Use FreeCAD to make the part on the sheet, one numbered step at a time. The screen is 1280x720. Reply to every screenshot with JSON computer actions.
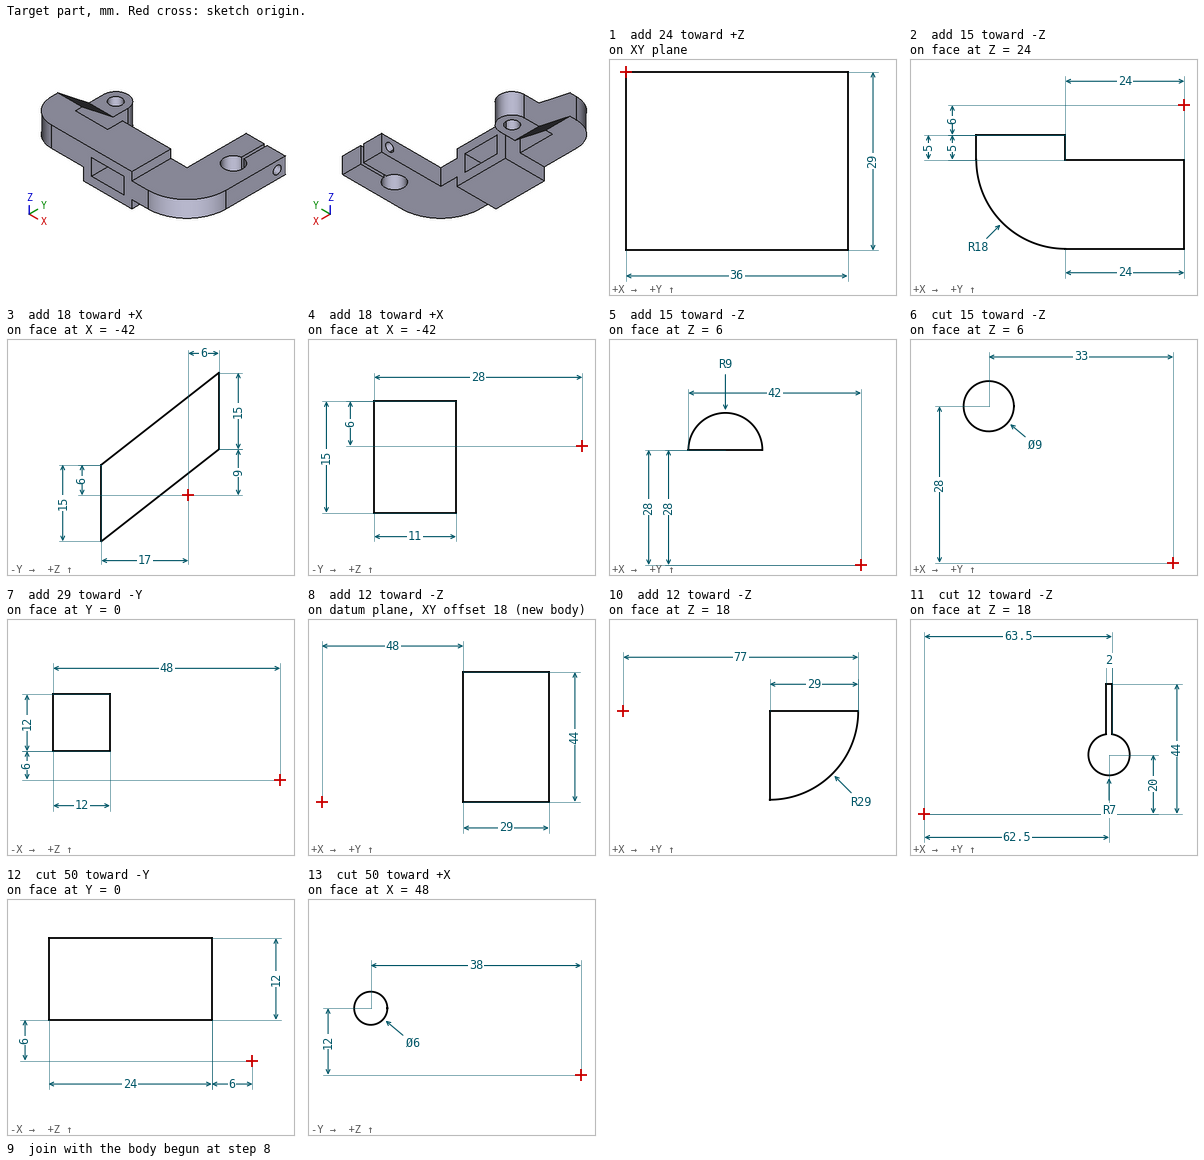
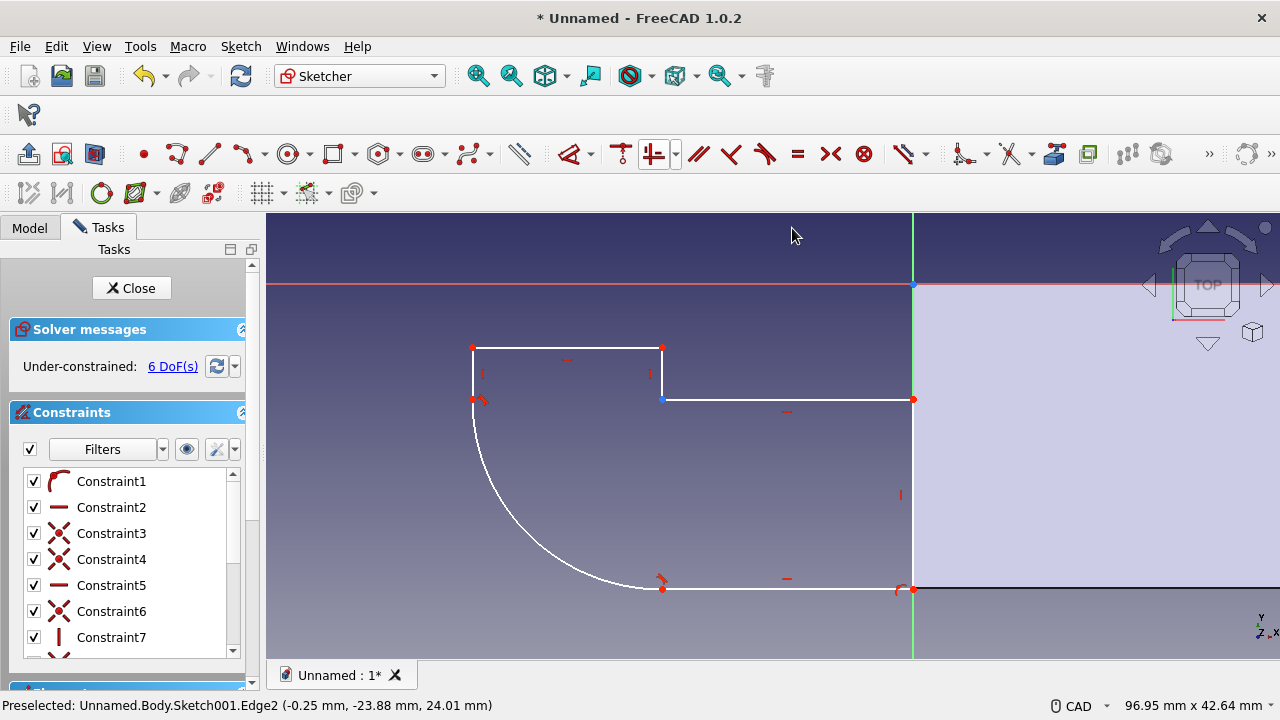
{"action": "left_click", "coordinate": [493, 486]}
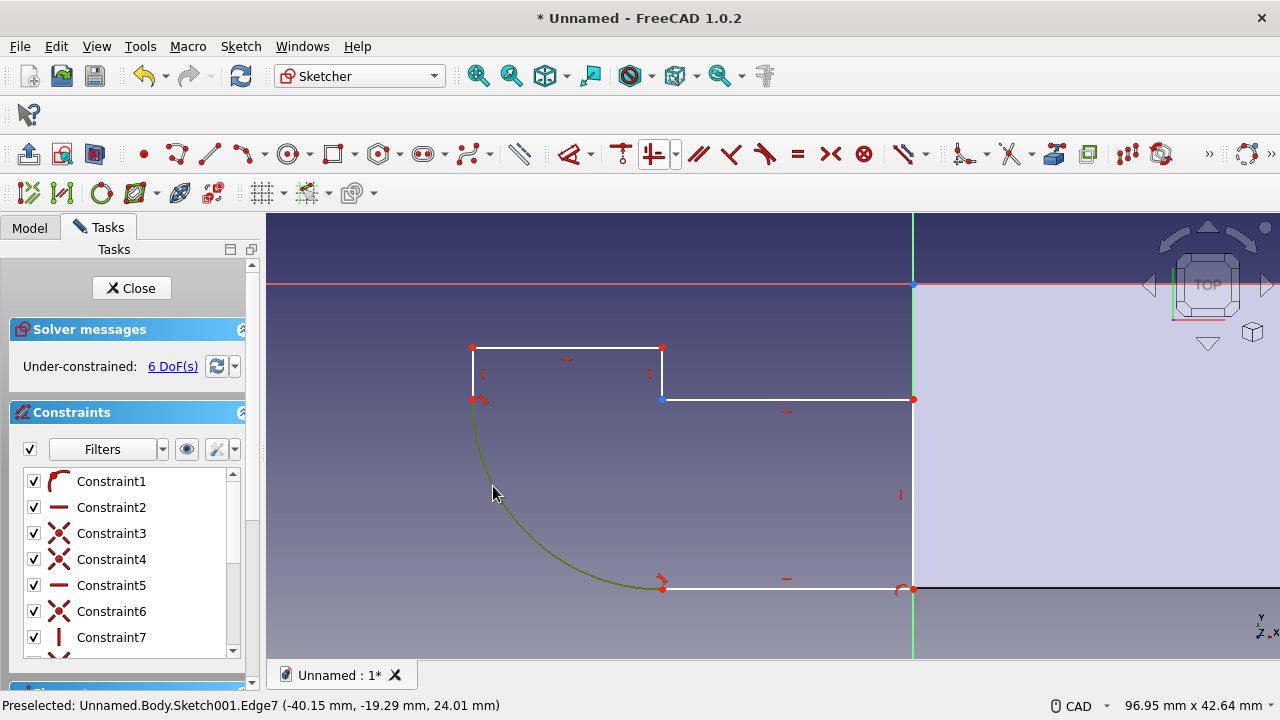
{"action": "key", "text": "k r"}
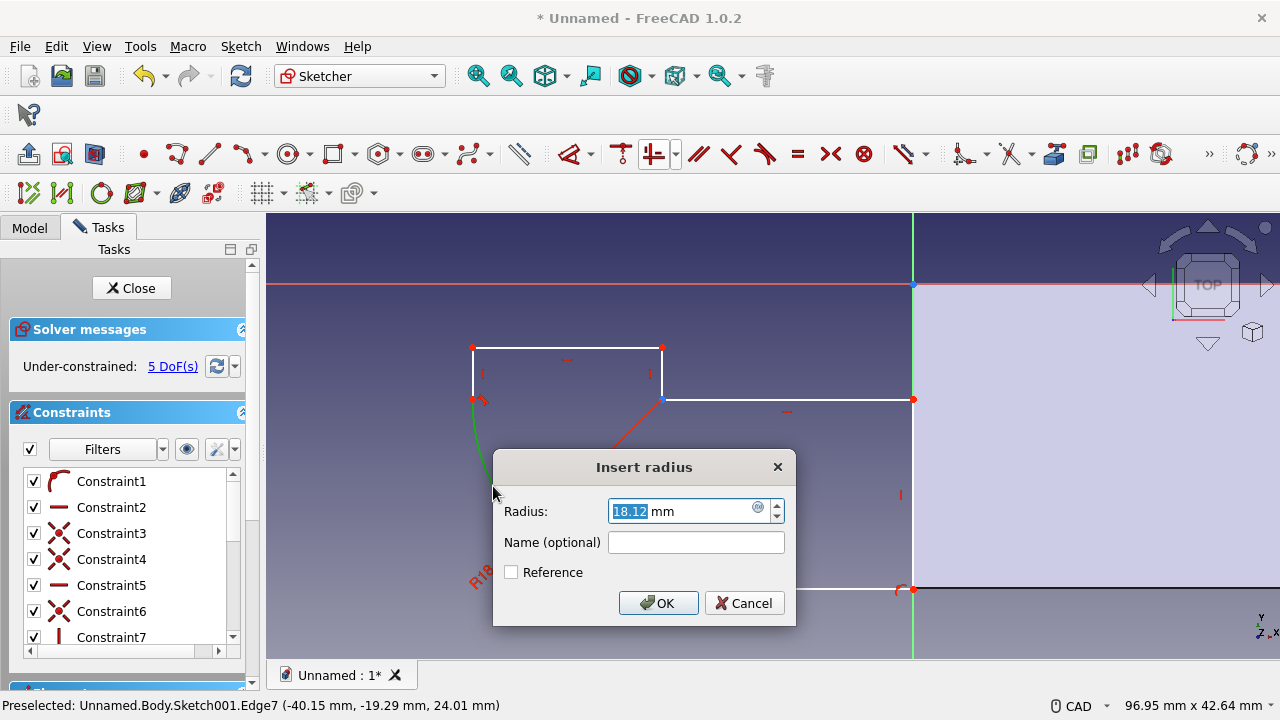
{"action": "type", "text": "18"}
{"action": "key", "text": "Return"}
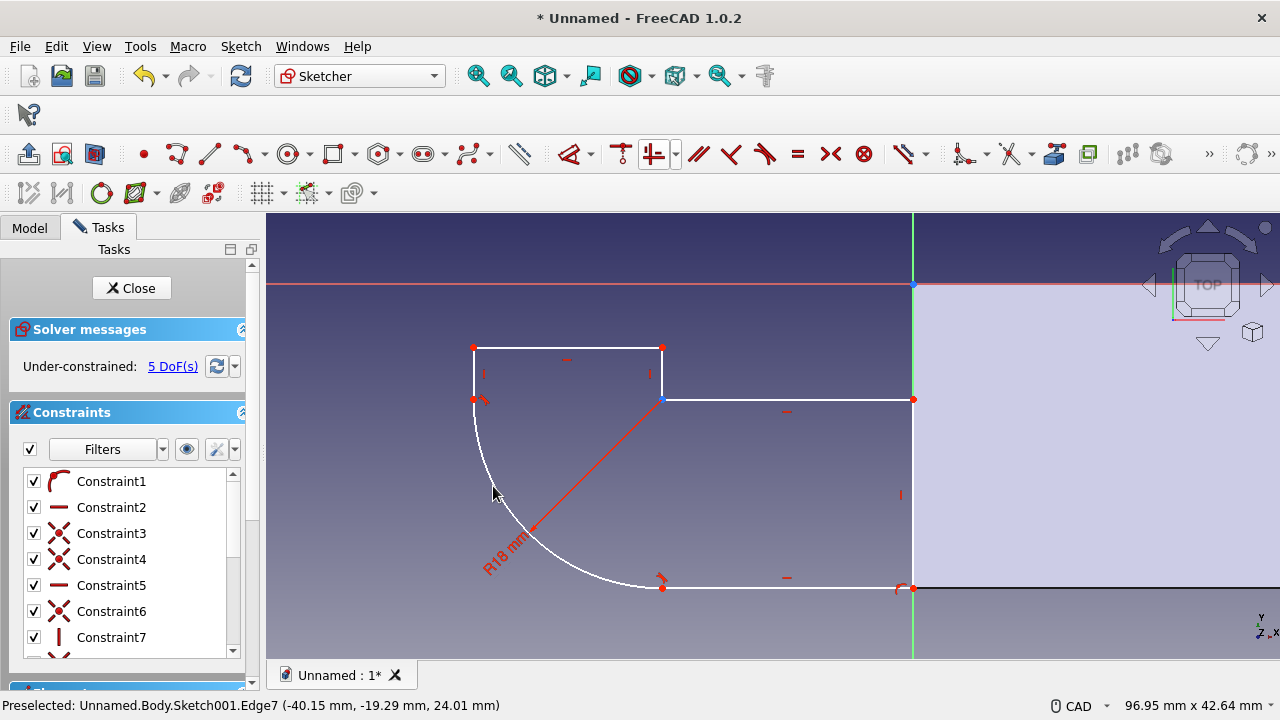
{"action": "left_click", "coordinate": [662, 384]}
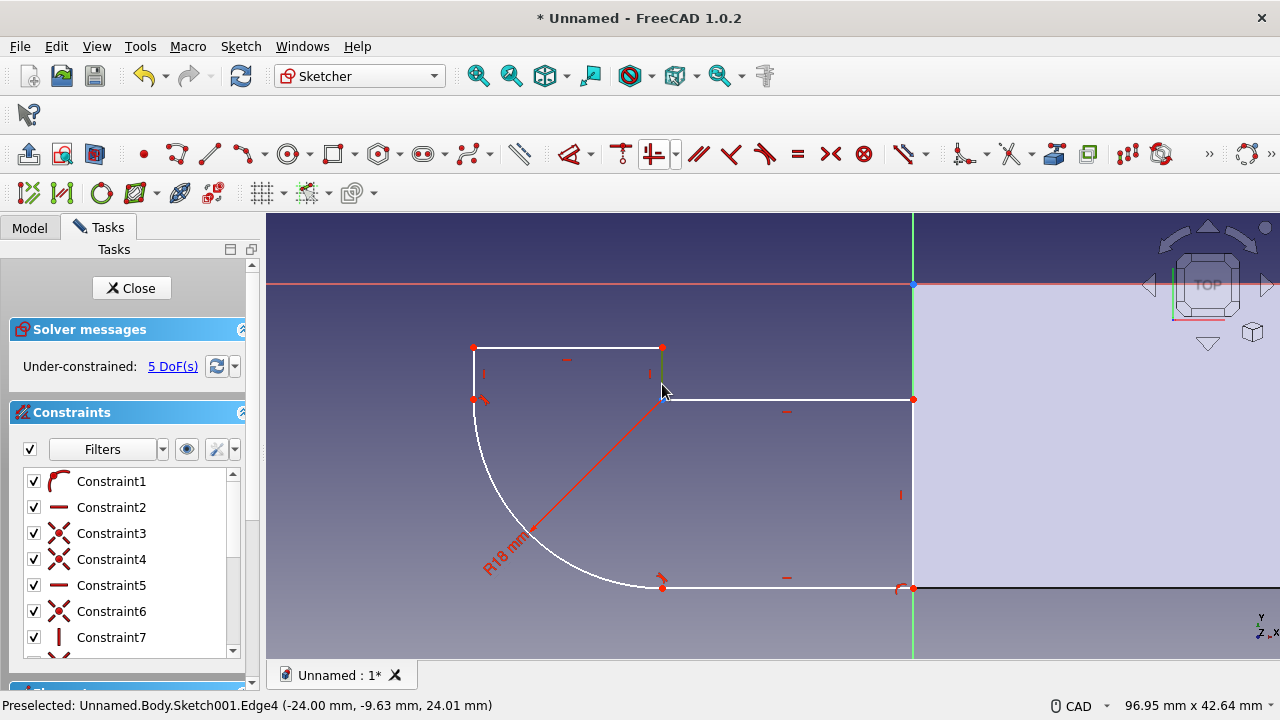
{"action": "key", "text": "i"}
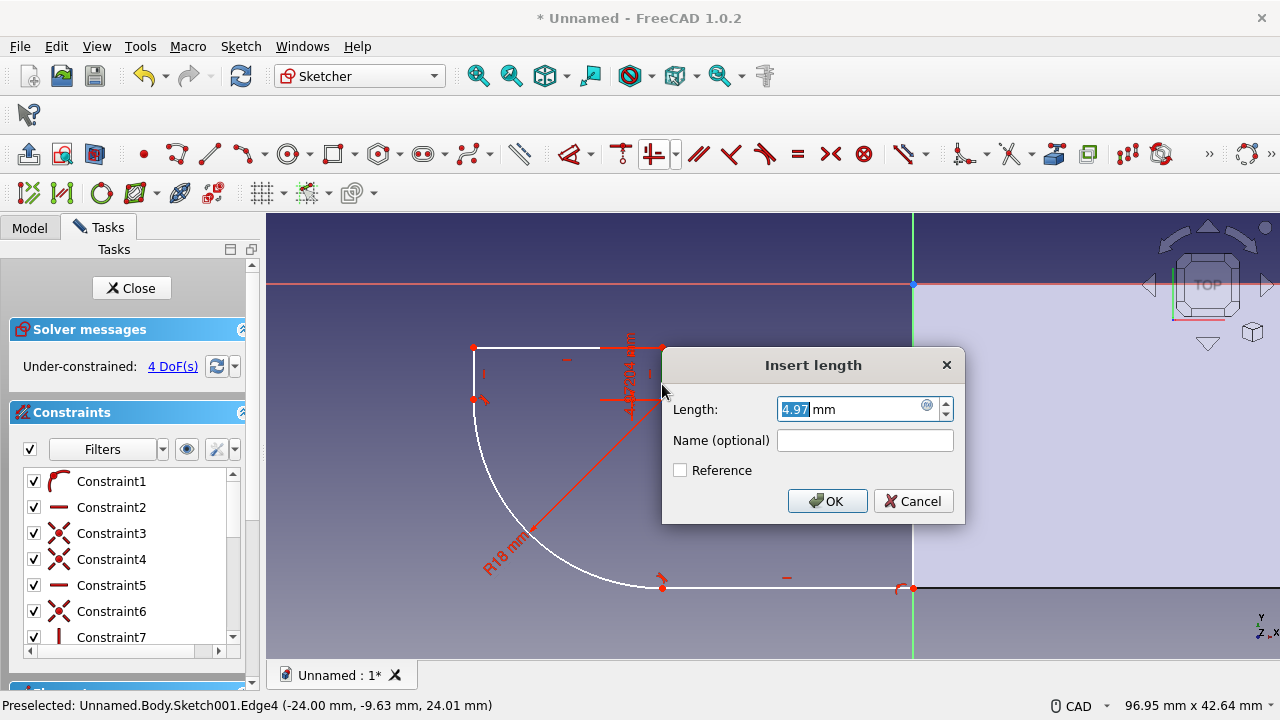
{"action": "type", "text": "5"}
{"action": "key", "text": "Return"}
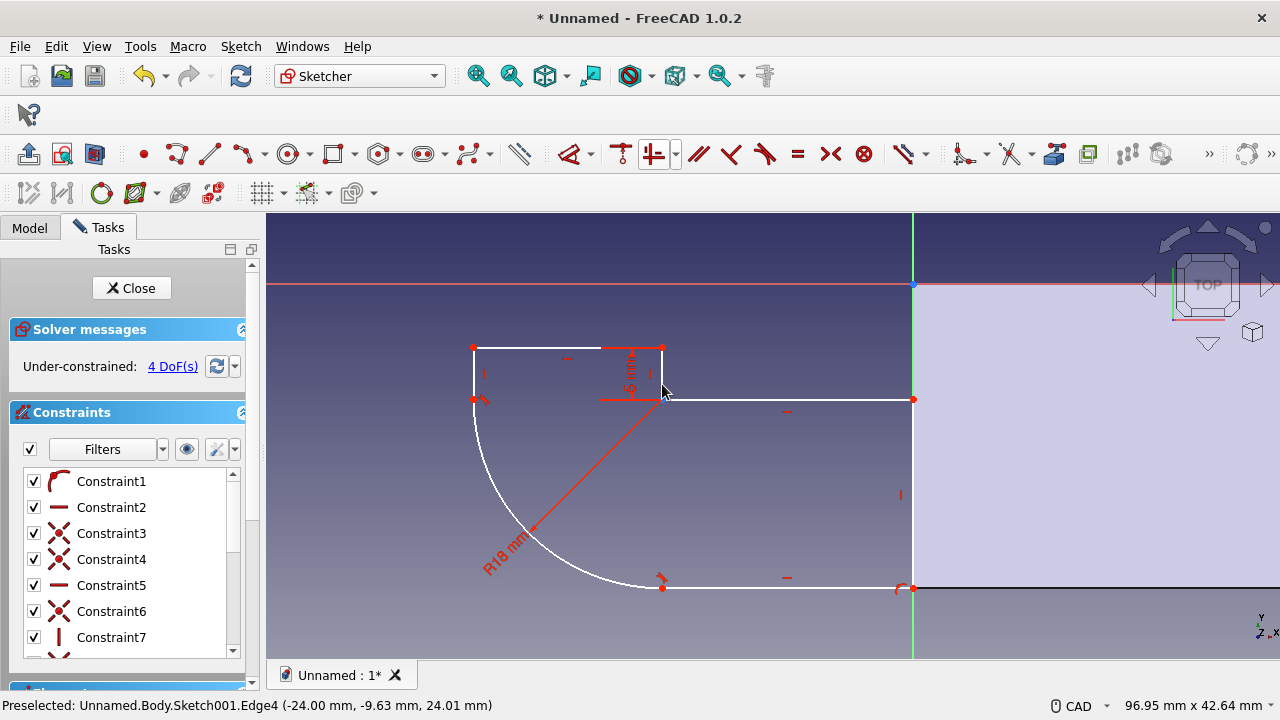
{"action": "left_click", "coordinate": [474, 363]}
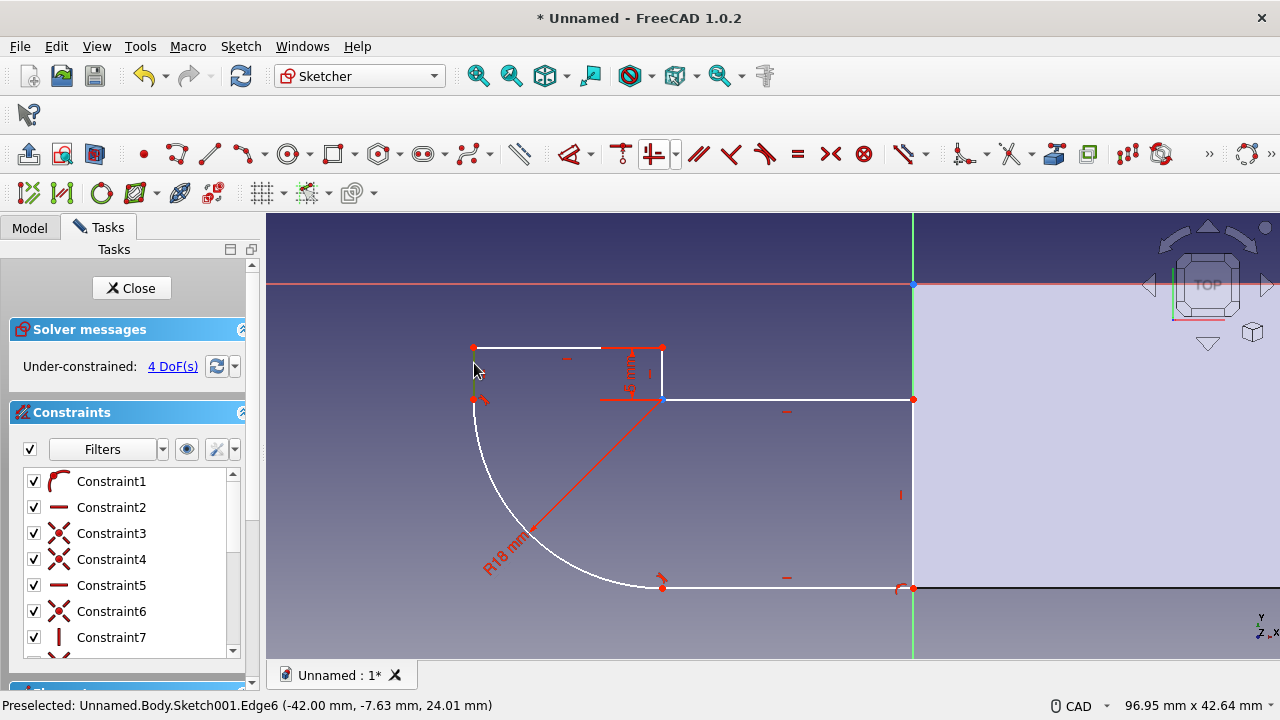
{"action": "key", "text": "i"}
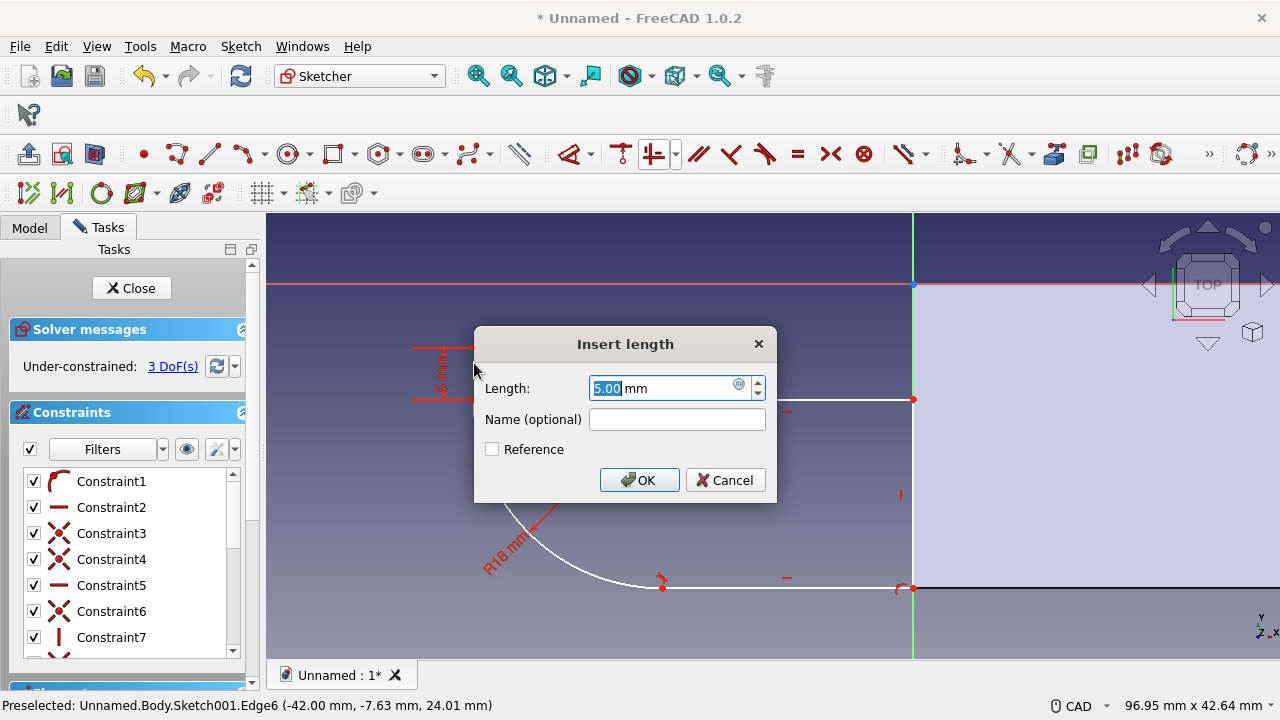
{"action": "type", "text": "5"}
{"action": "key", "text": "Return"}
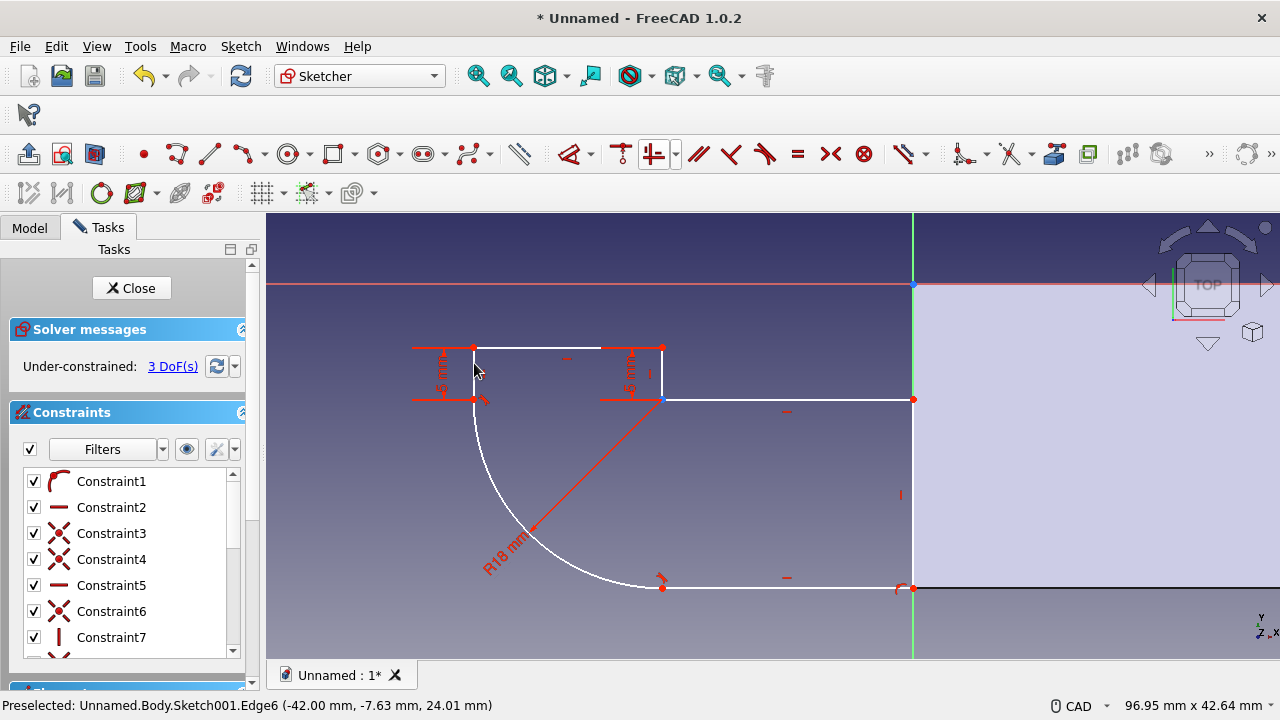
{"action": "left_click", "coordinate": [737, 588]}